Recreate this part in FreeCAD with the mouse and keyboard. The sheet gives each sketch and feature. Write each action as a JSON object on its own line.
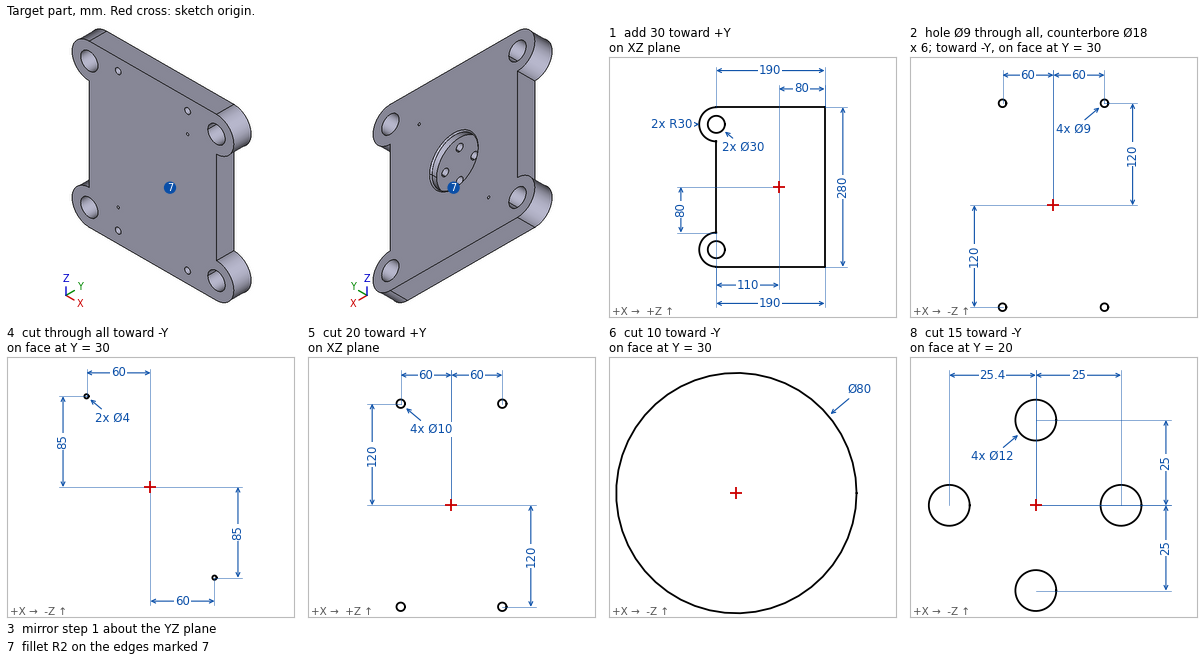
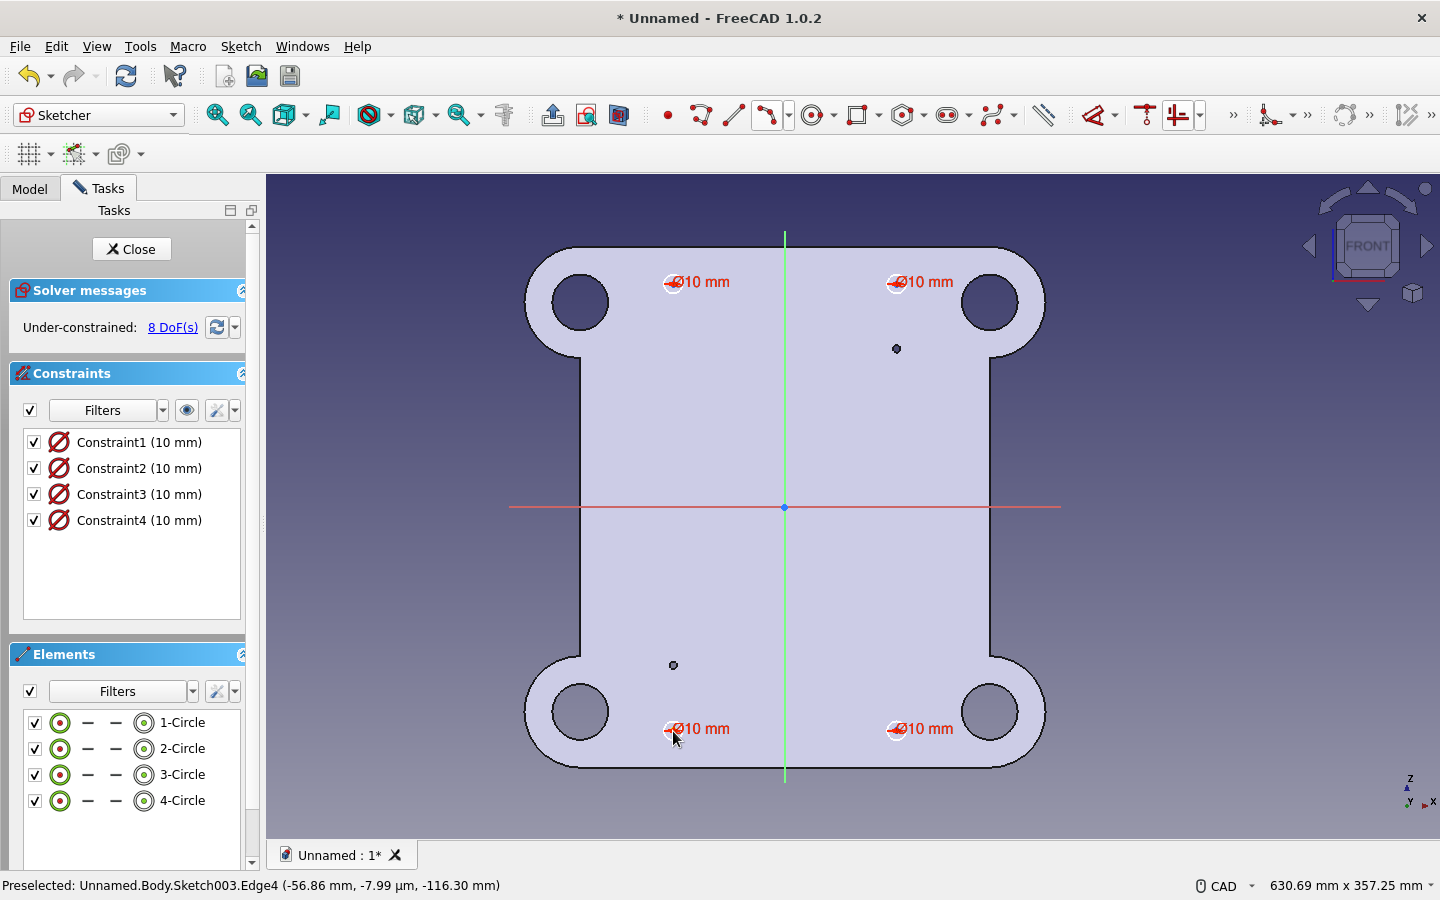
{"action": "left_click", "coordinate": [673, 284]}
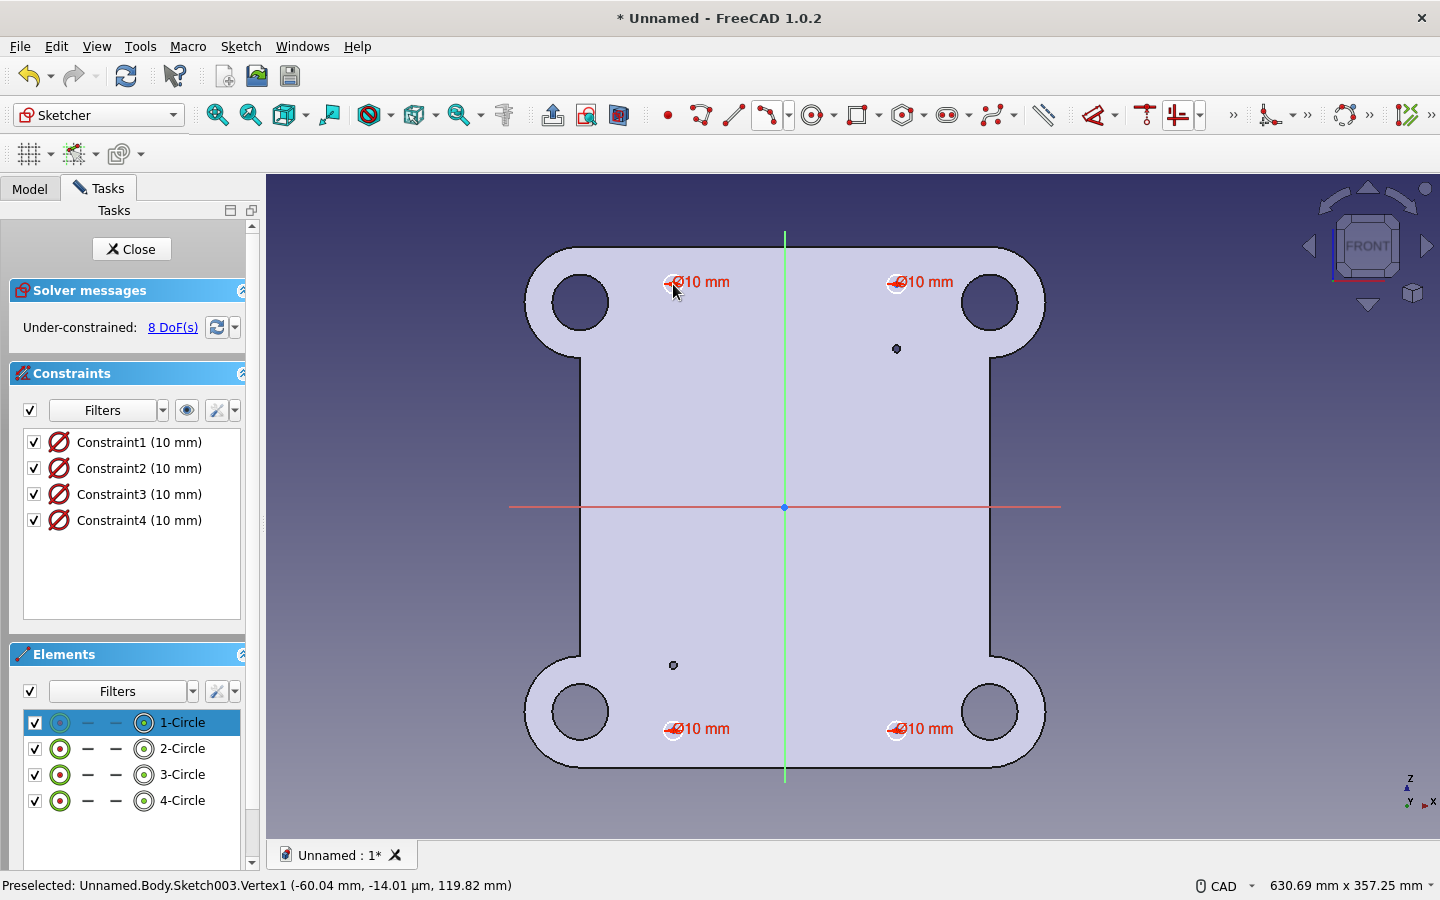
{"action": "left_click", "coordinate": [897, 284]}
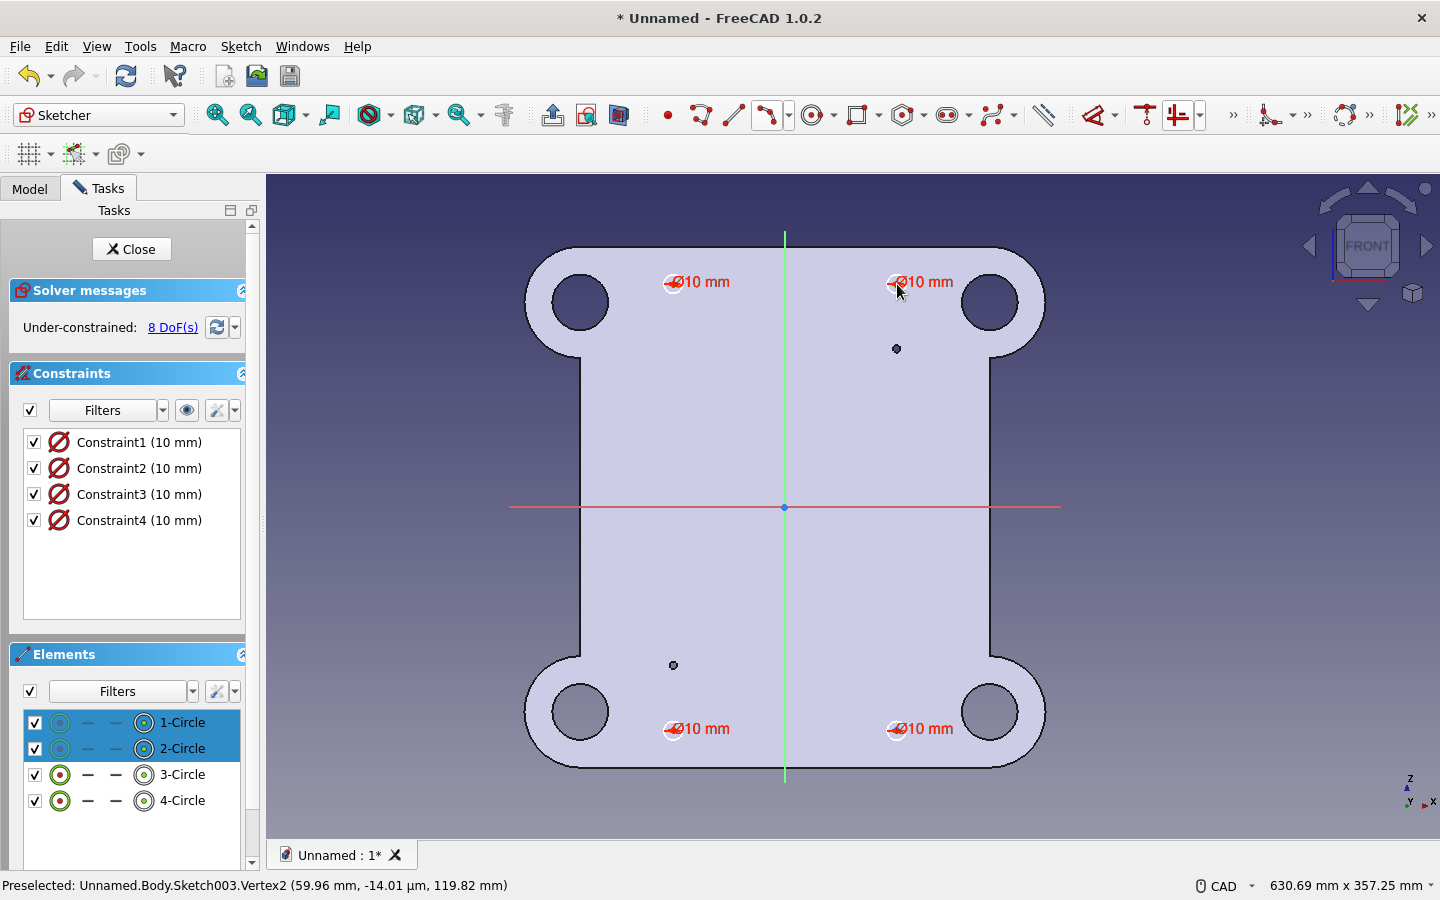
{"action": "key", "text": "h"}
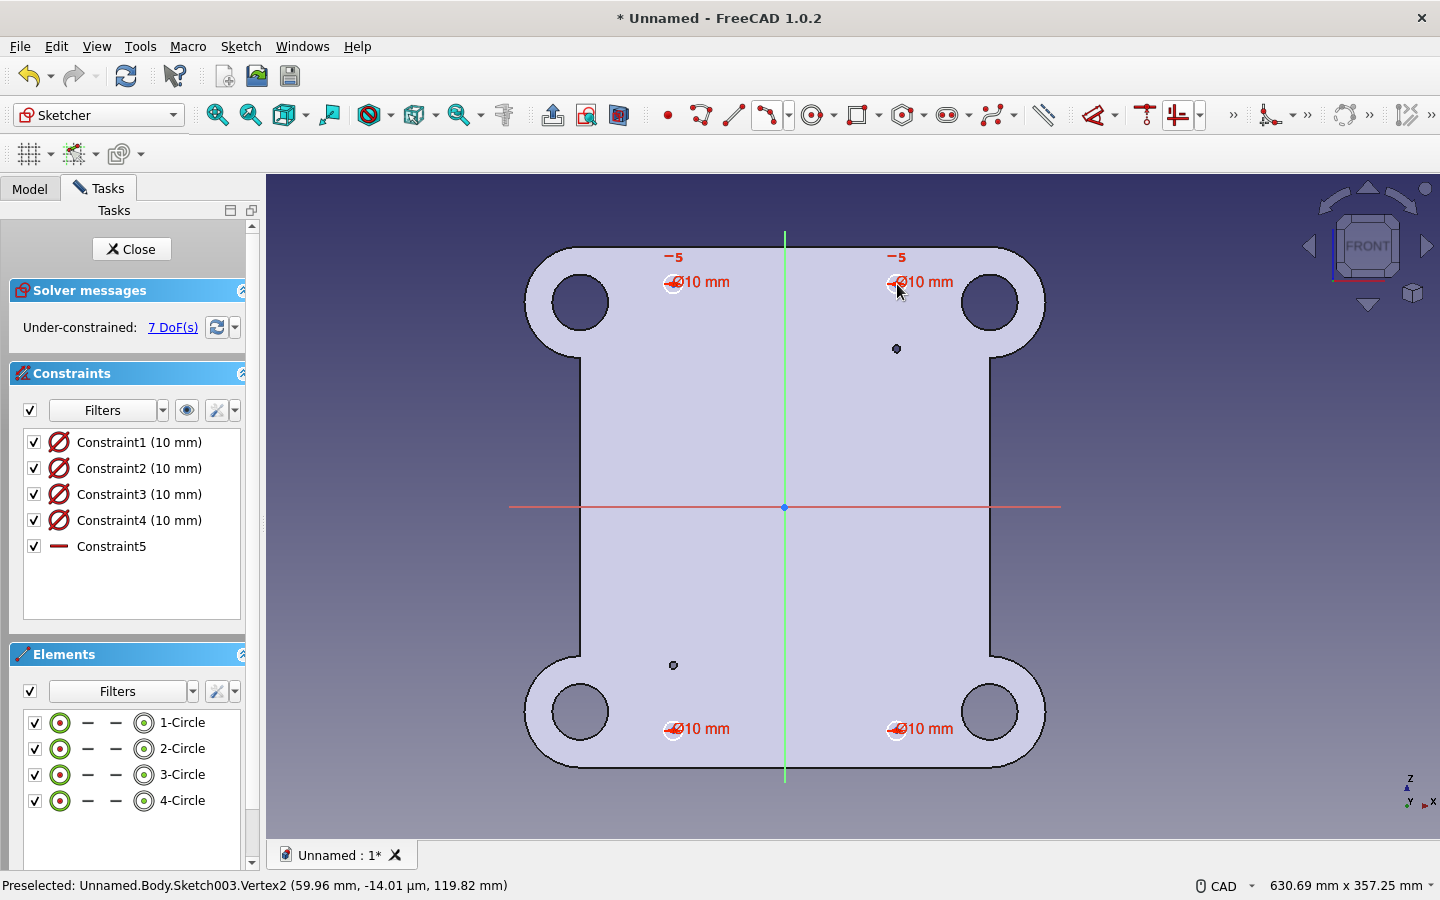
{"action": "left_click", "coordinate": [897, 284]}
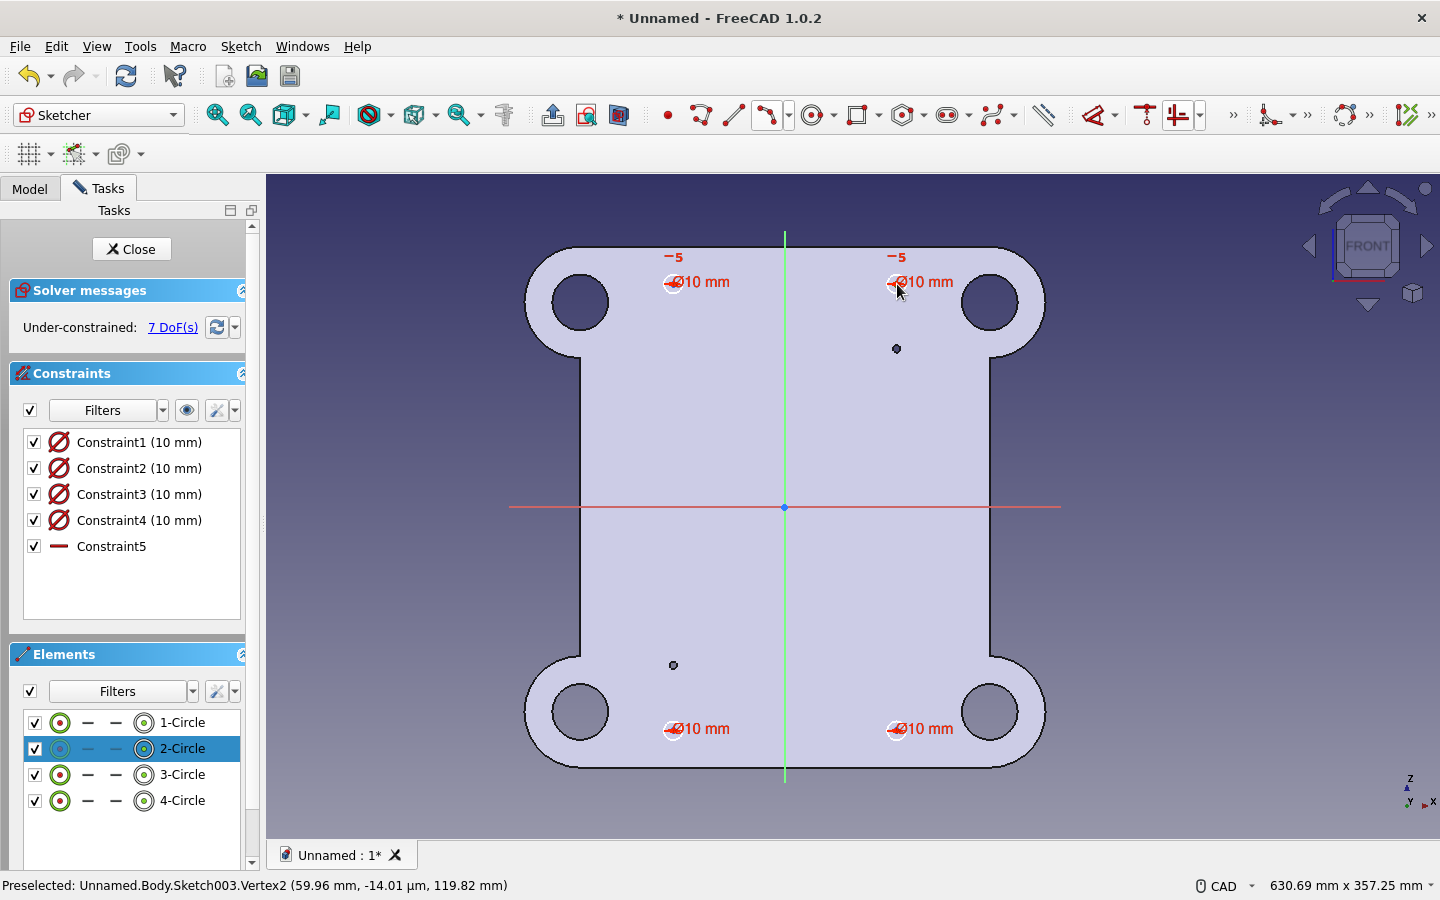
{"action": "left_click", "coordinate": [897, 731]}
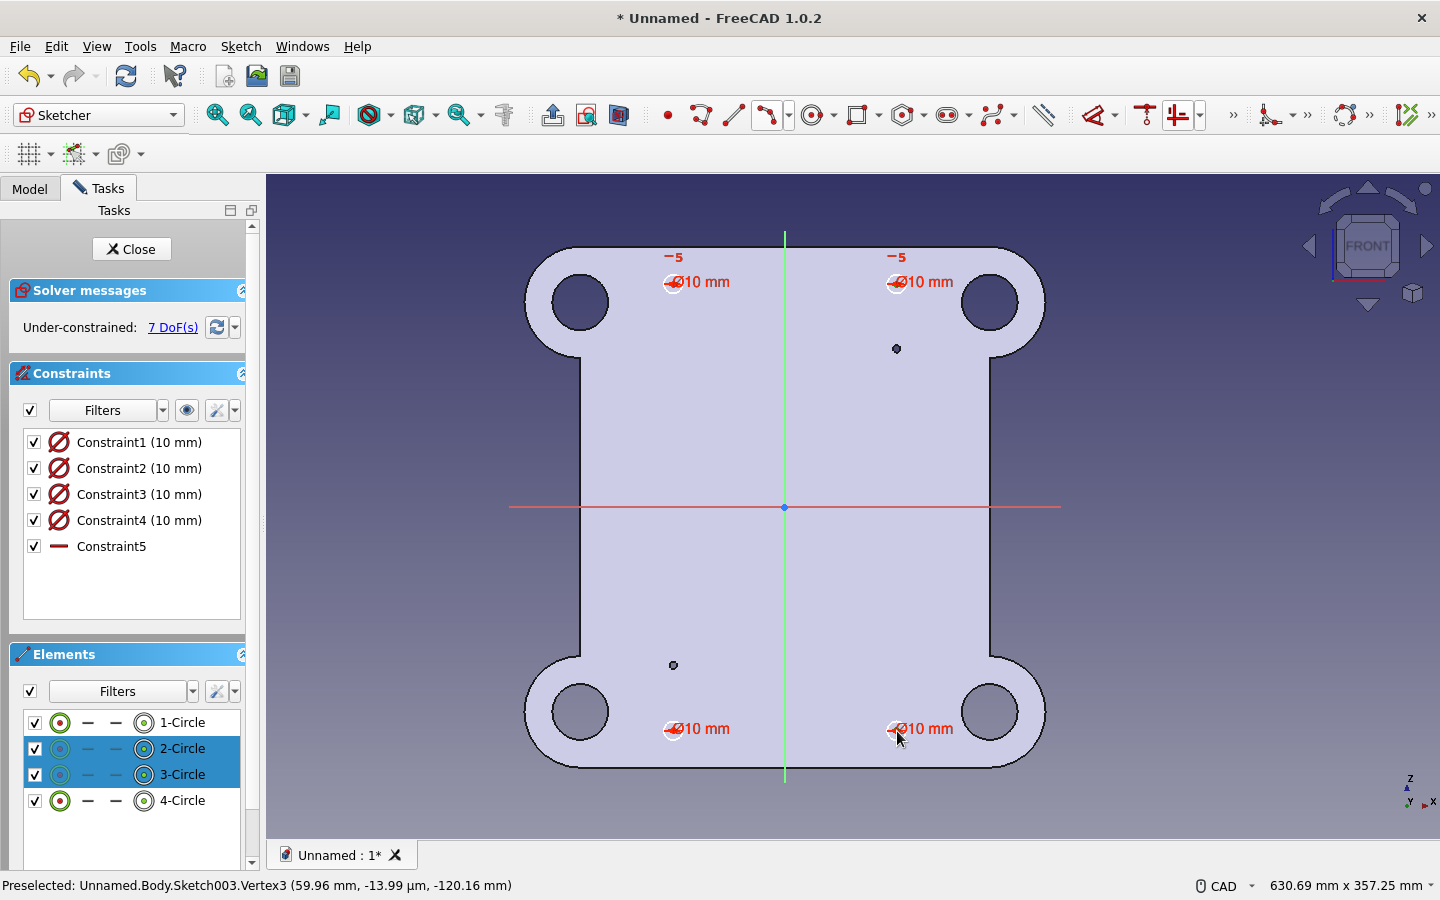
{"action": "left_click", "coordinate": [1200, 116]}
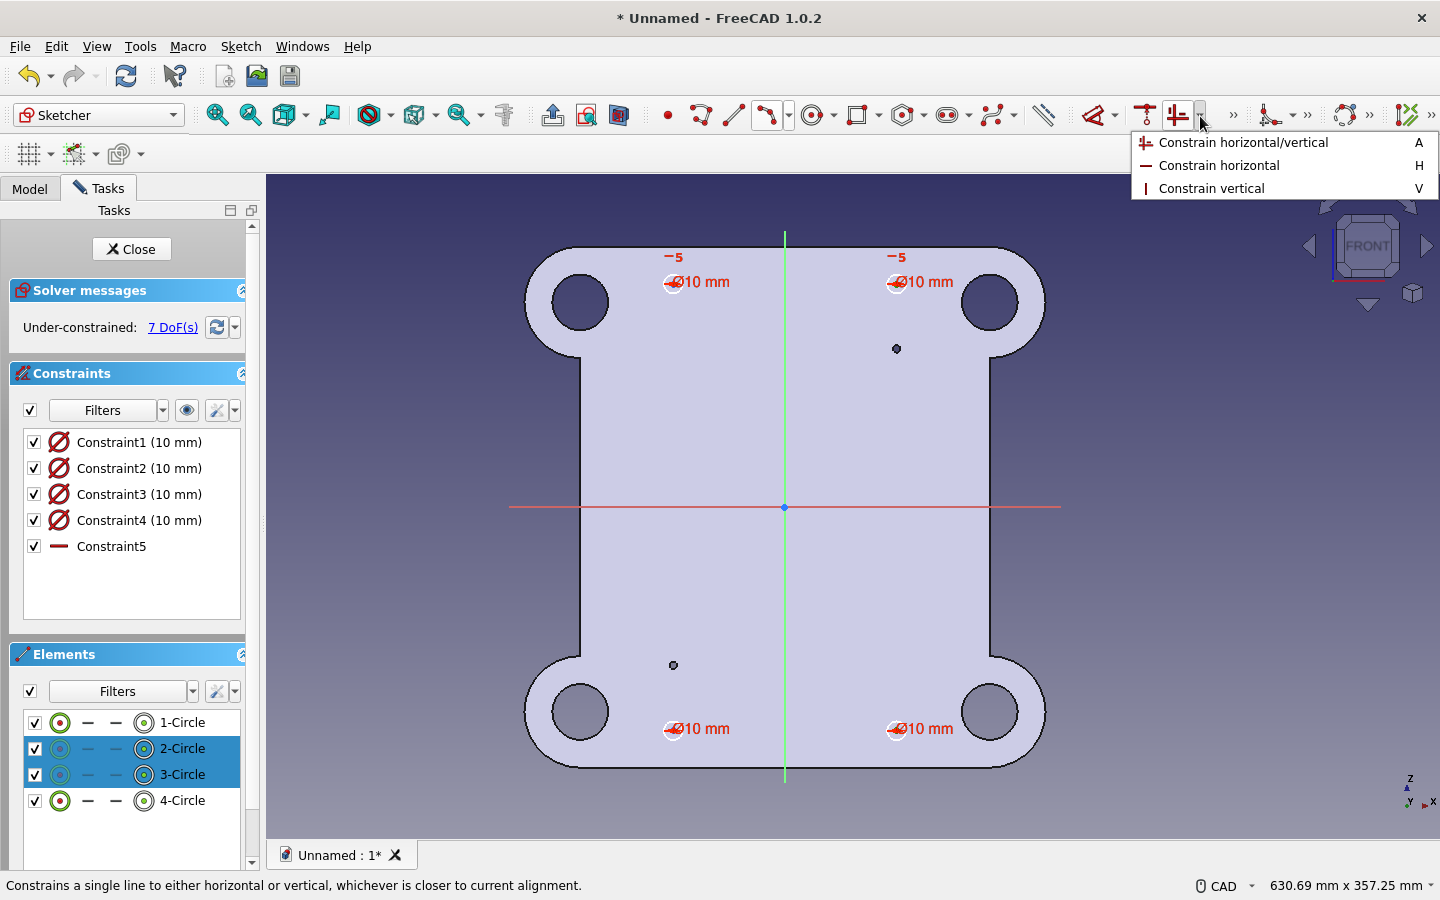
{"action": "left_click", "coordinate": [1285, 188]}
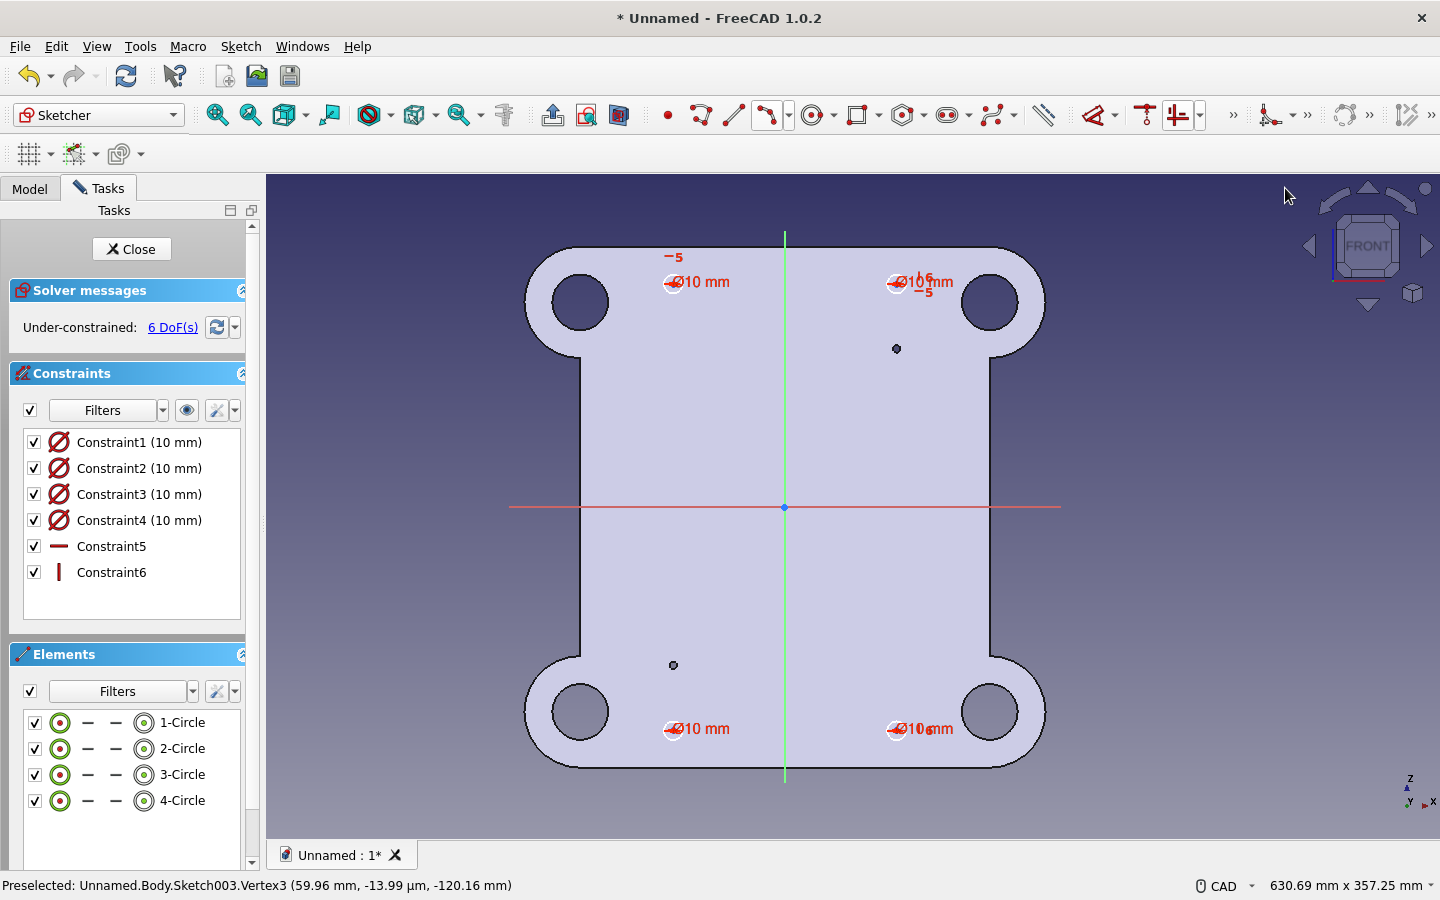
{"action": "left_click", "coordinate": [673, 284]}